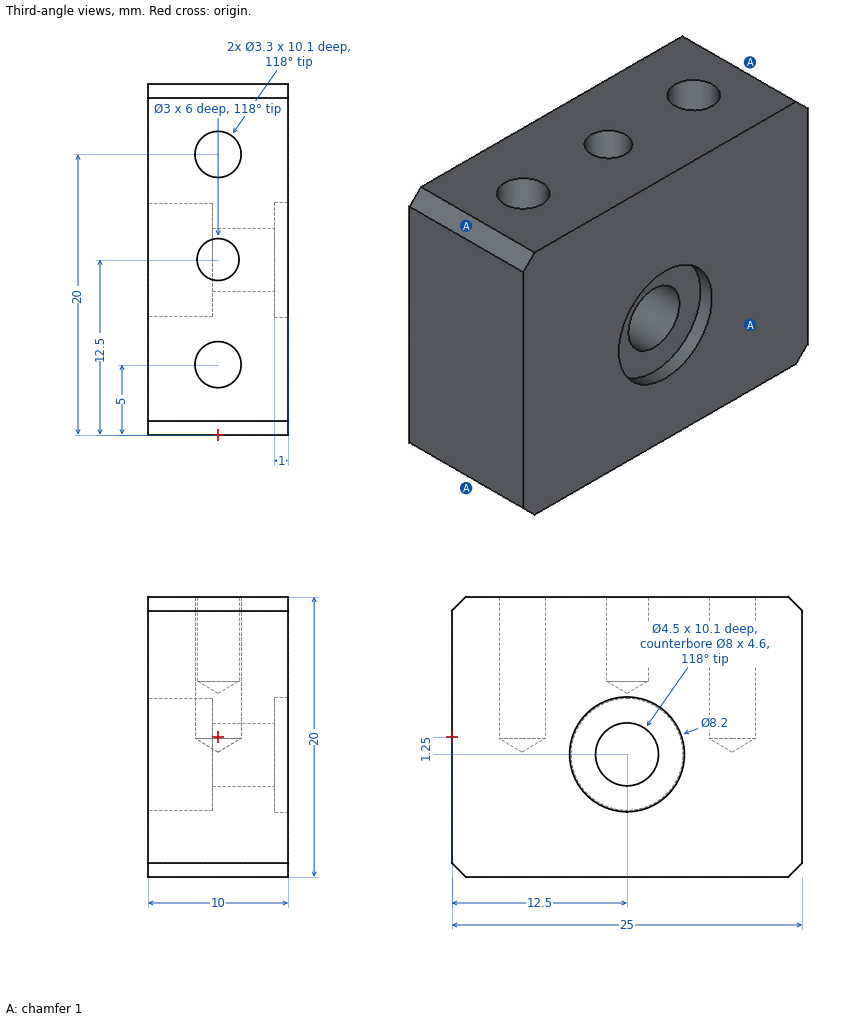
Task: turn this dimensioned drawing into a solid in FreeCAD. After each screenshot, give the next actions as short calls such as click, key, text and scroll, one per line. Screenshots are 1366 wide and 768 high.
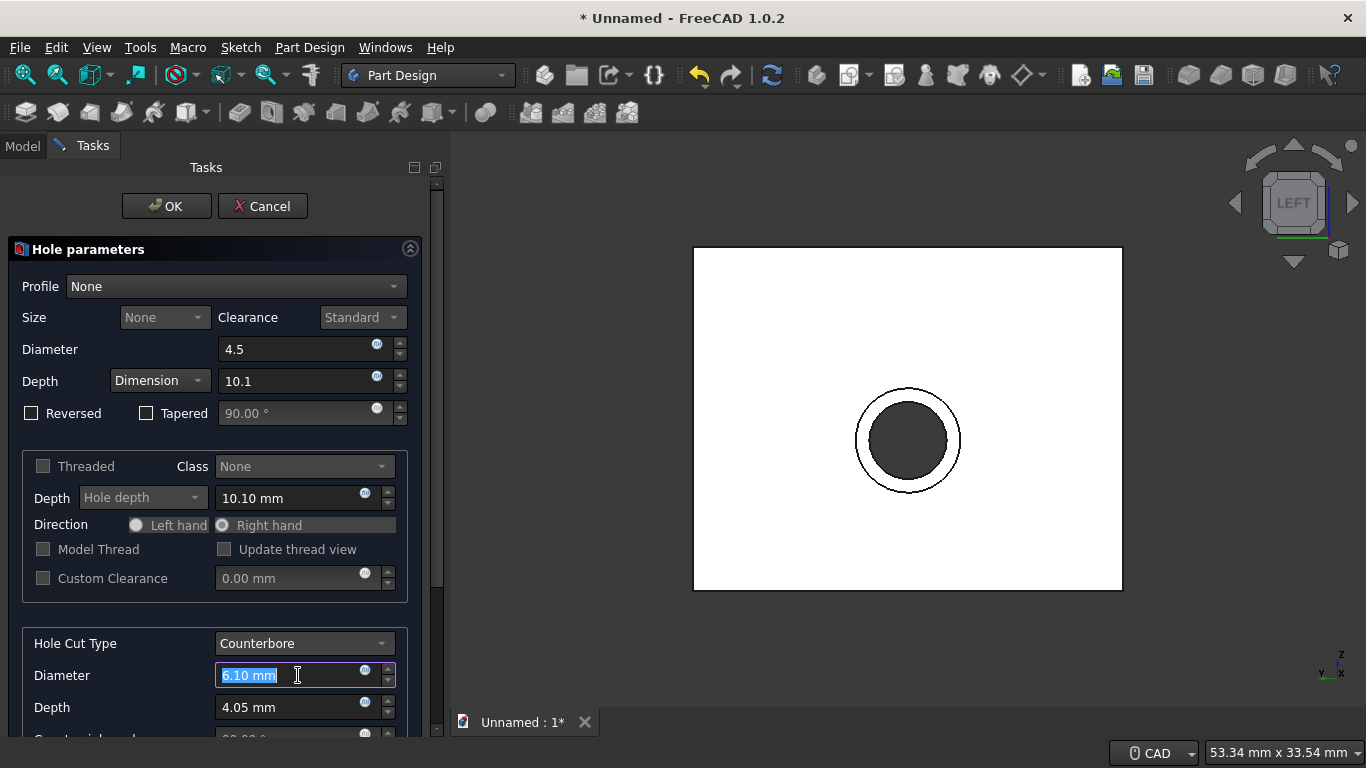
text(8)
key(Tab)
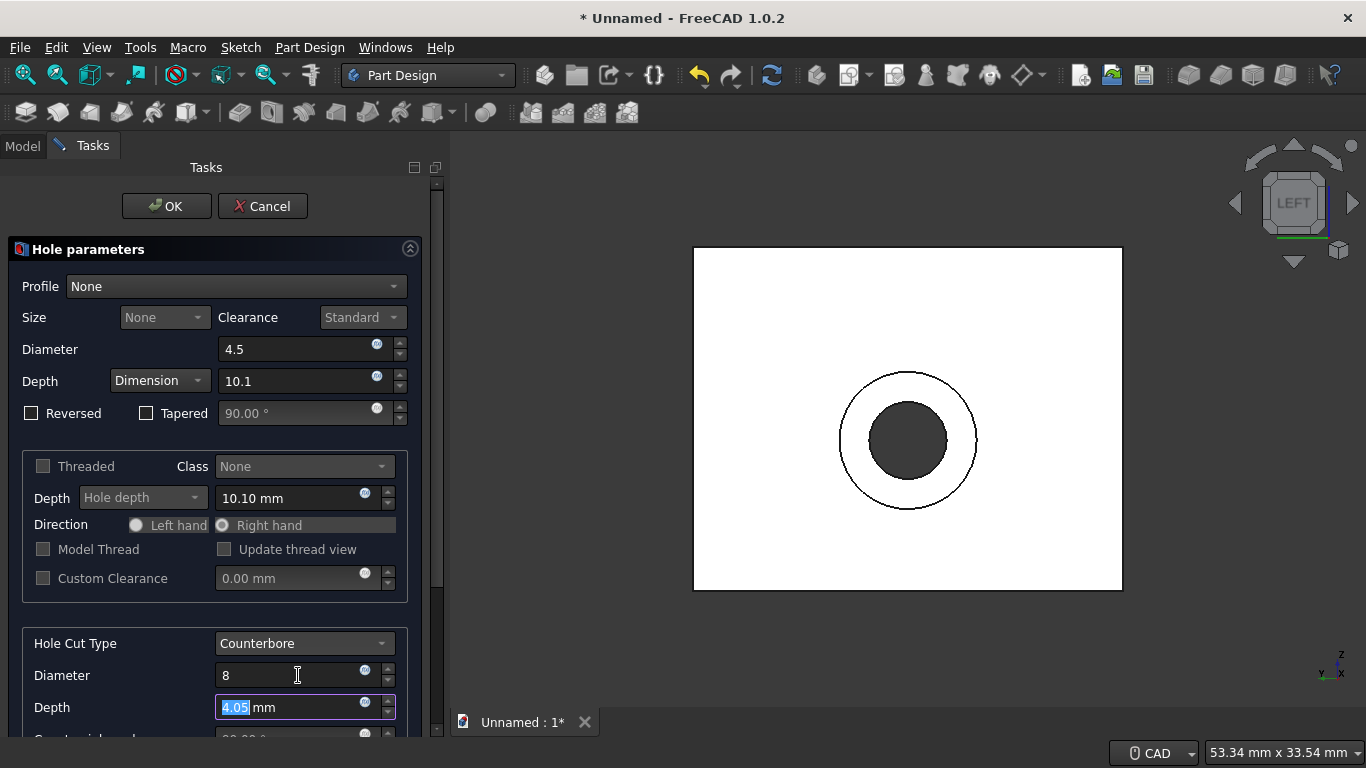
text(4.6)
key(Tab)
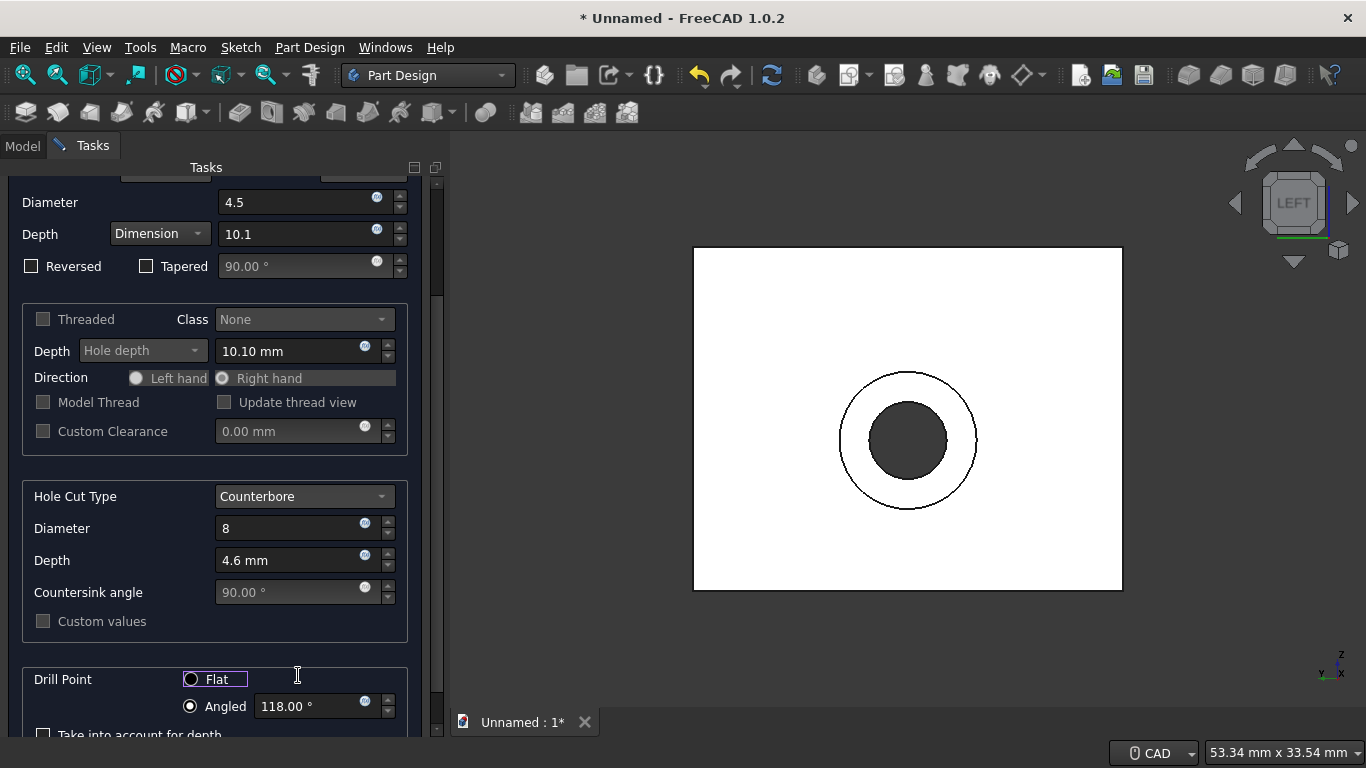
scroll(437, 456, up, 4)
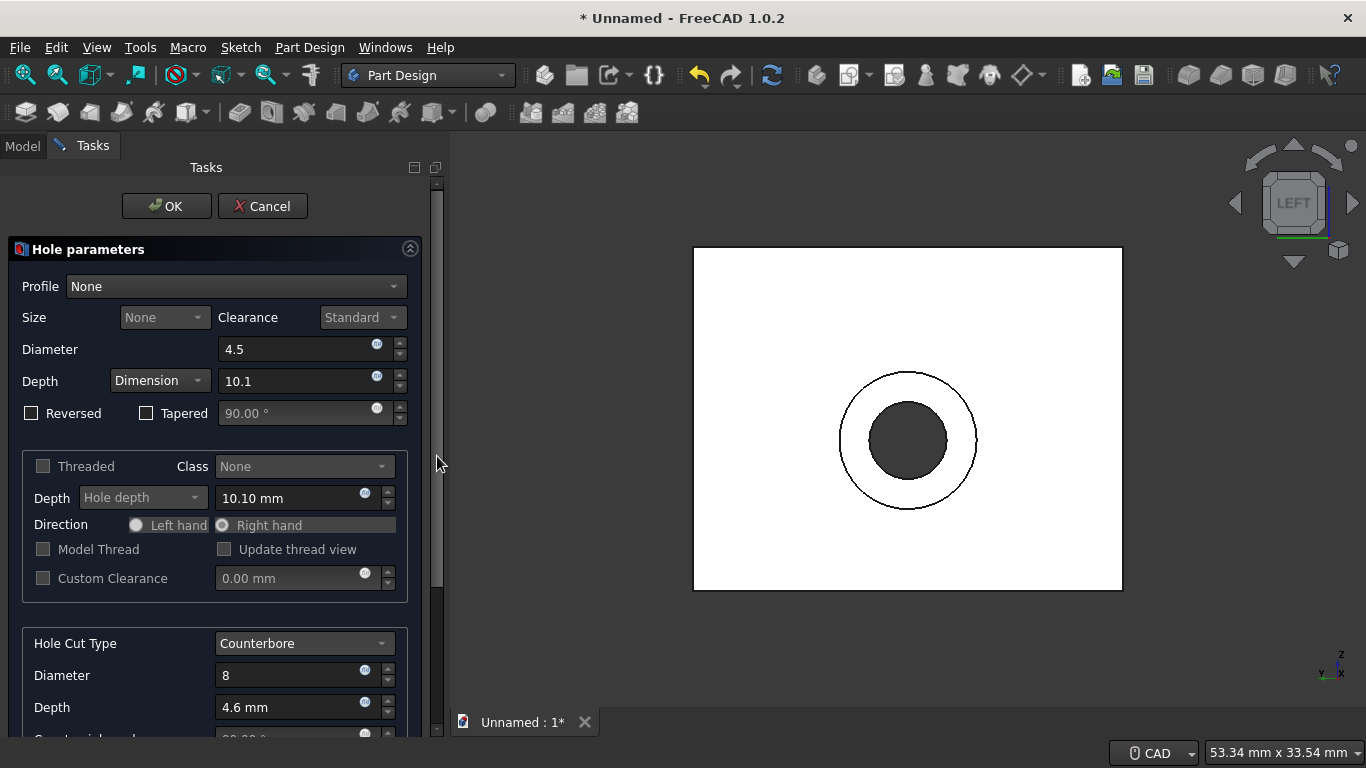
click(167, 206)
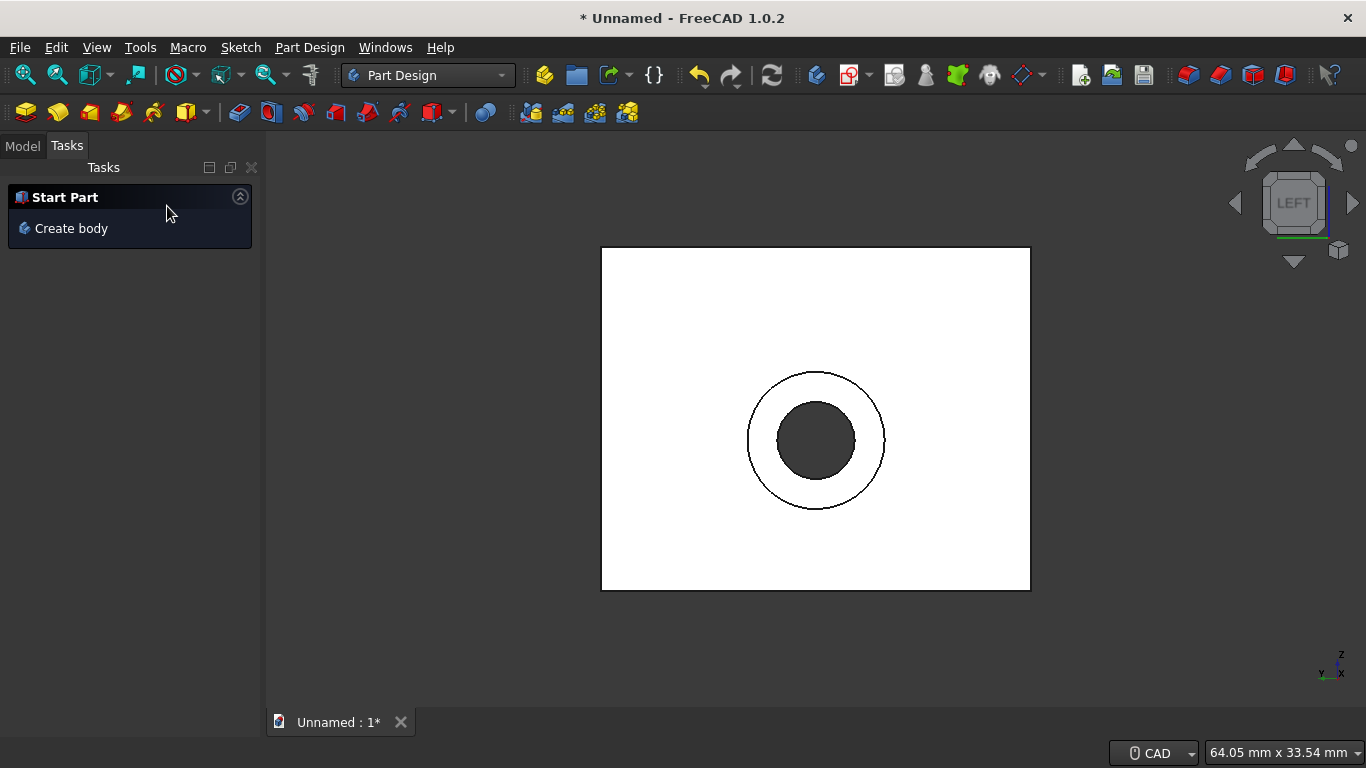
key(0)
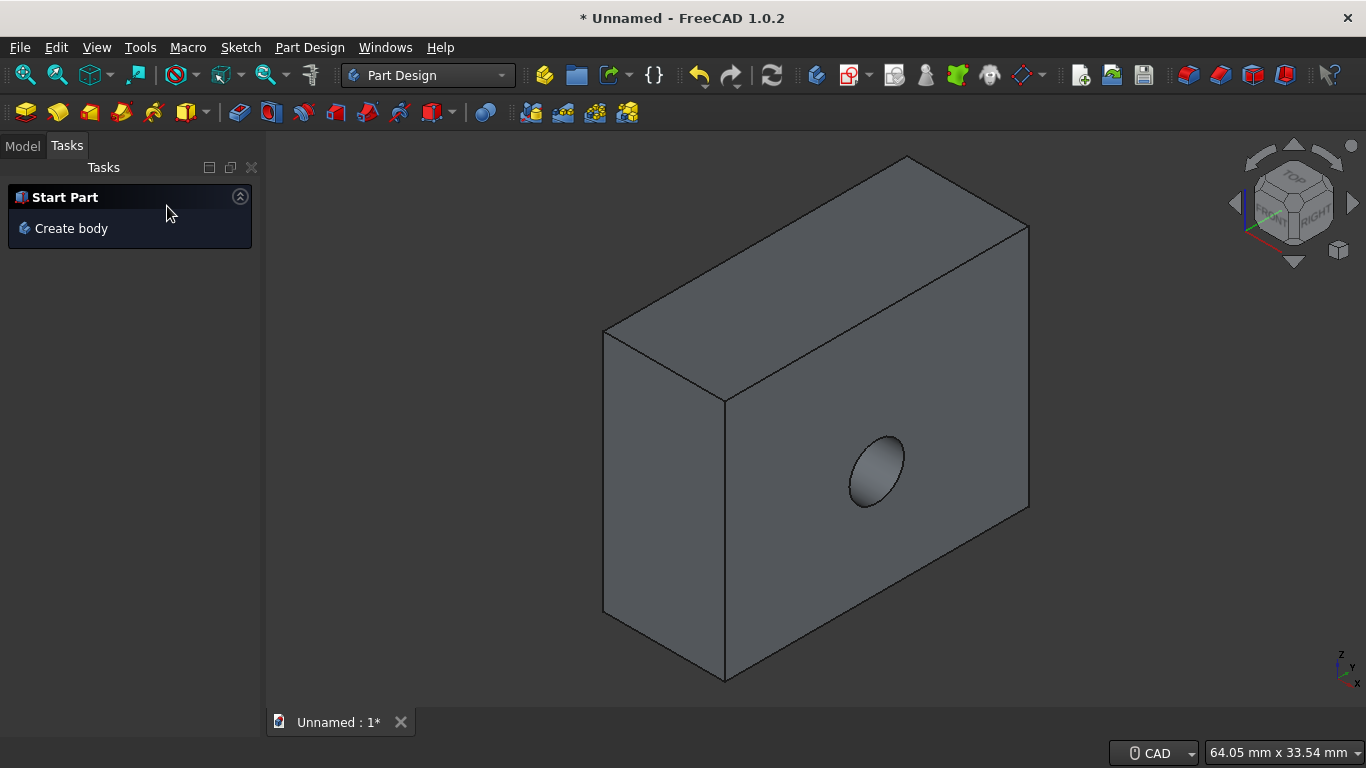
click(790, 463)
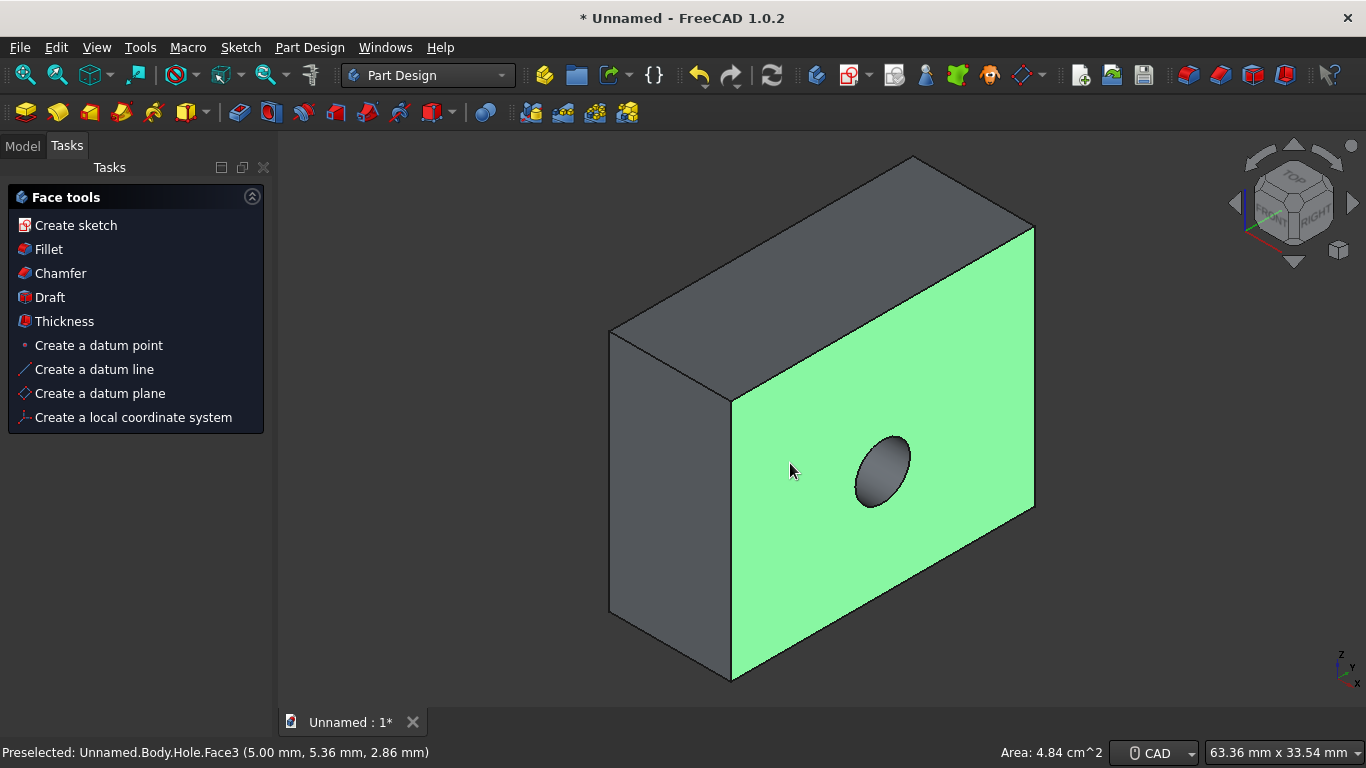
click(850, 76)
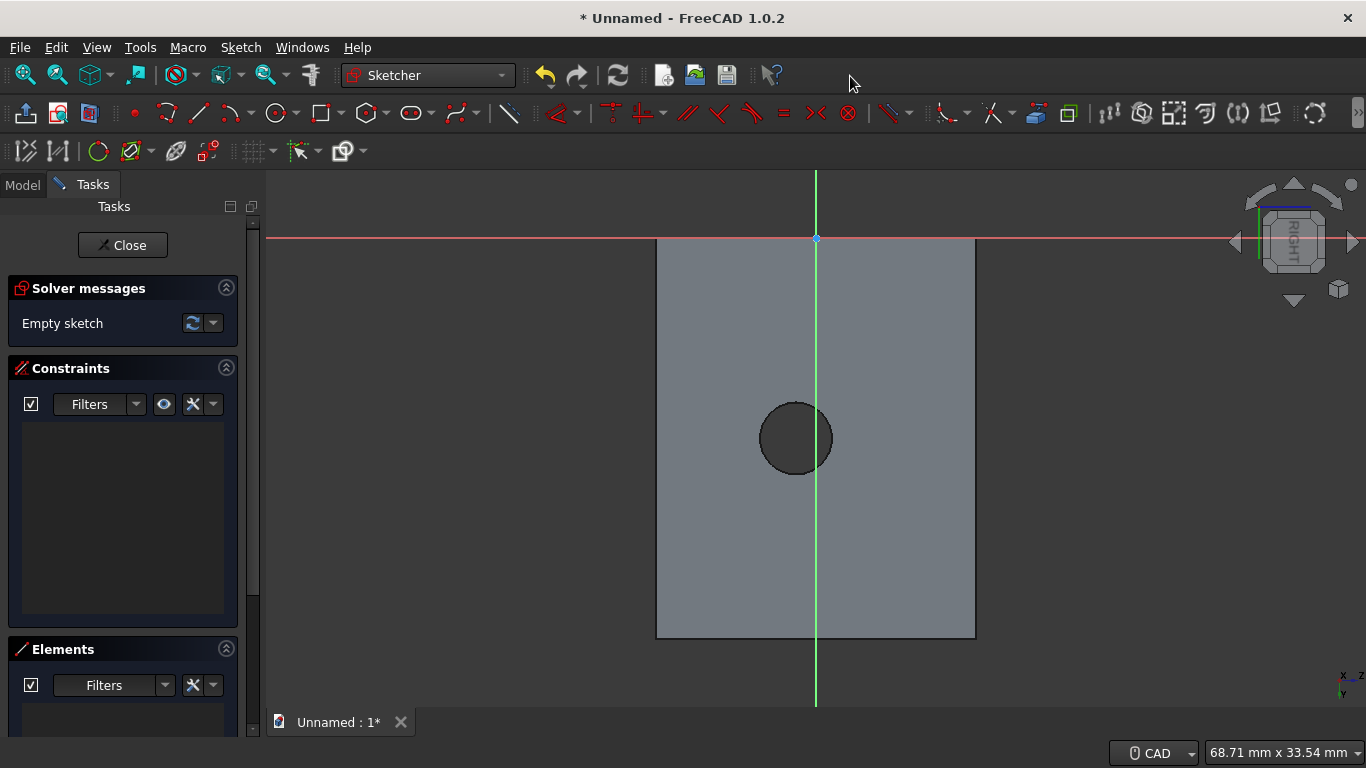
click(276, 114)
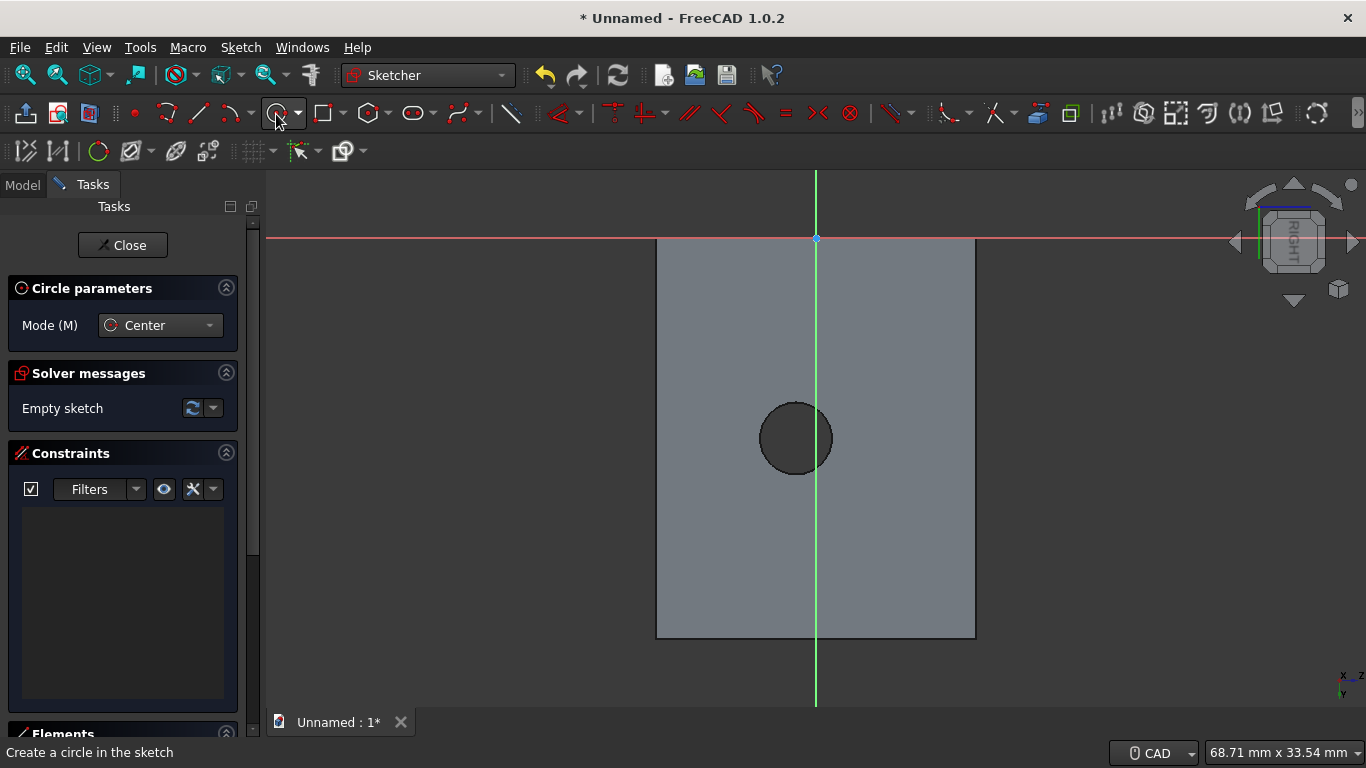
click(796, 438)
click(842, 392)
key(Escape)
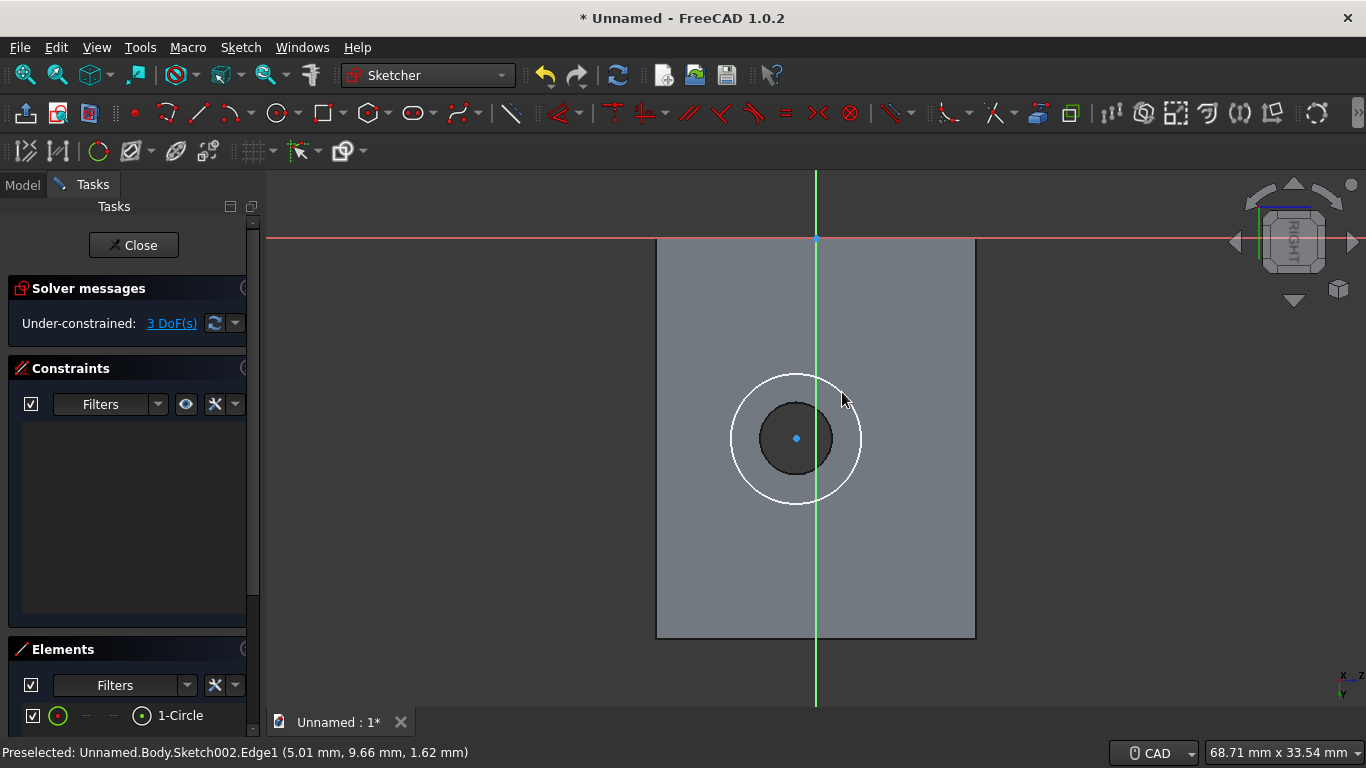
click(558, 114)